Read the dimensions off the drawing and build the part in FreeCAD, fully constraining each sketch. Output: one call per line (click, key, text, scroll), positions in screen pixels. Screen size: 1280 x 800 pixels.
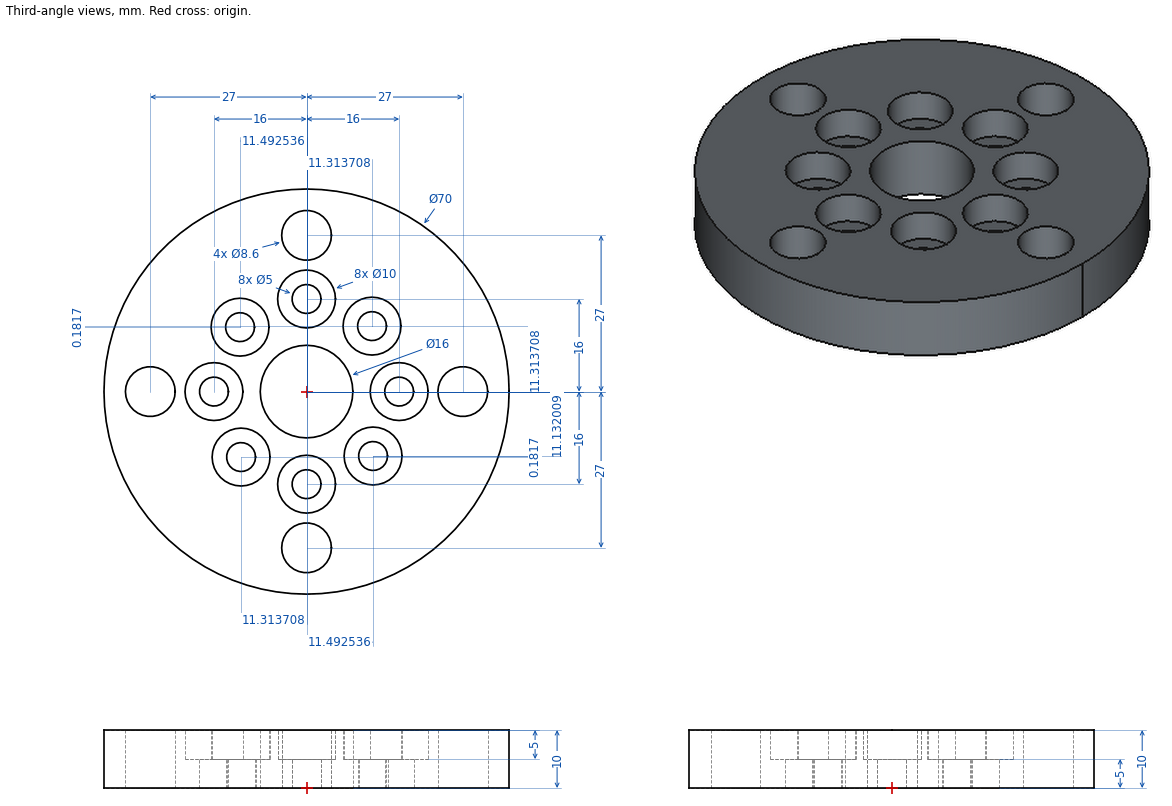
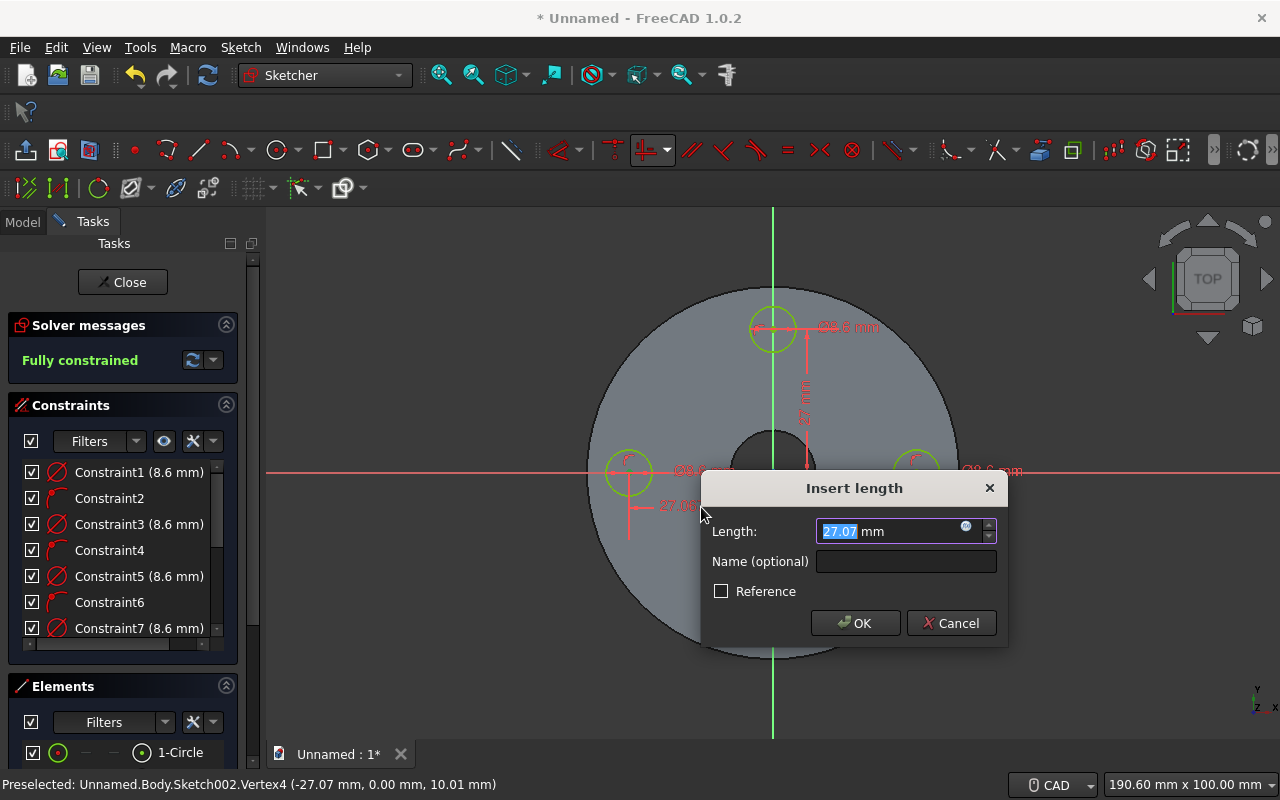
text(27)
key(Return)
key(Escape)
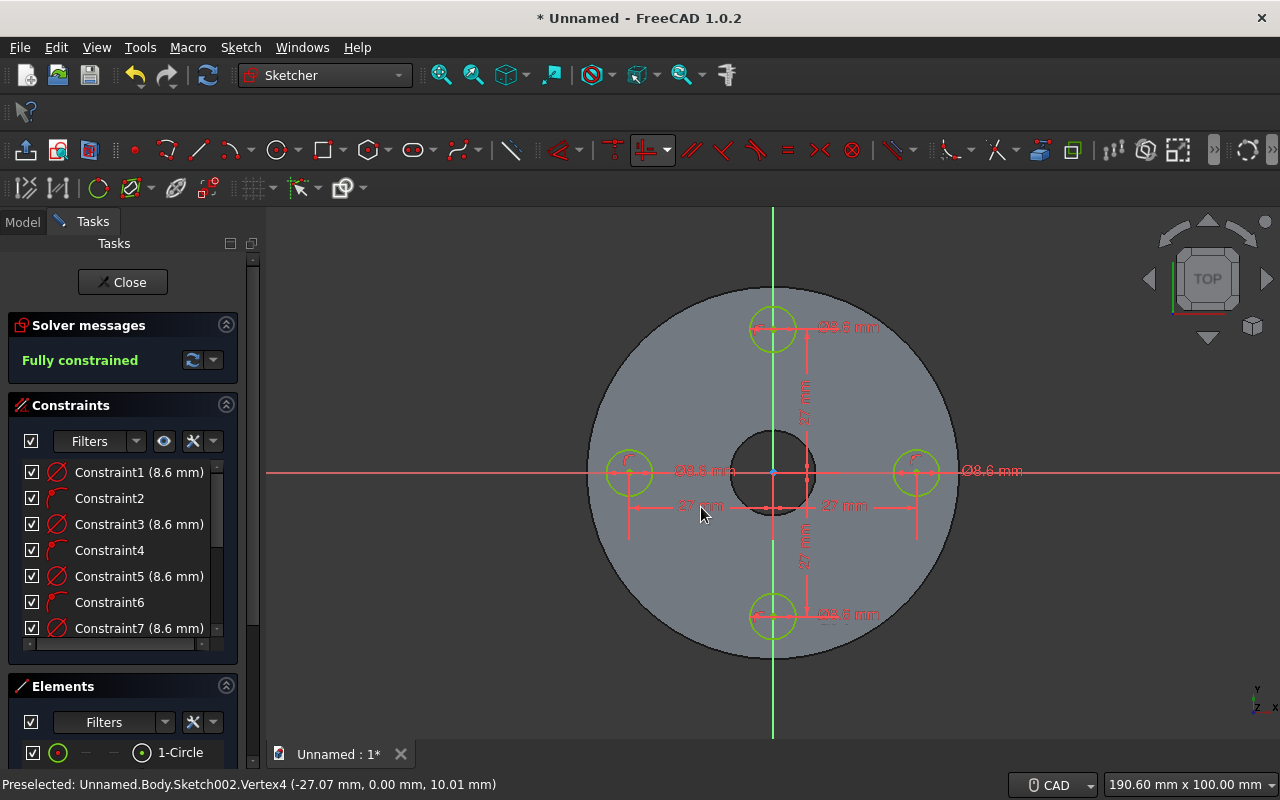
click(123, 282)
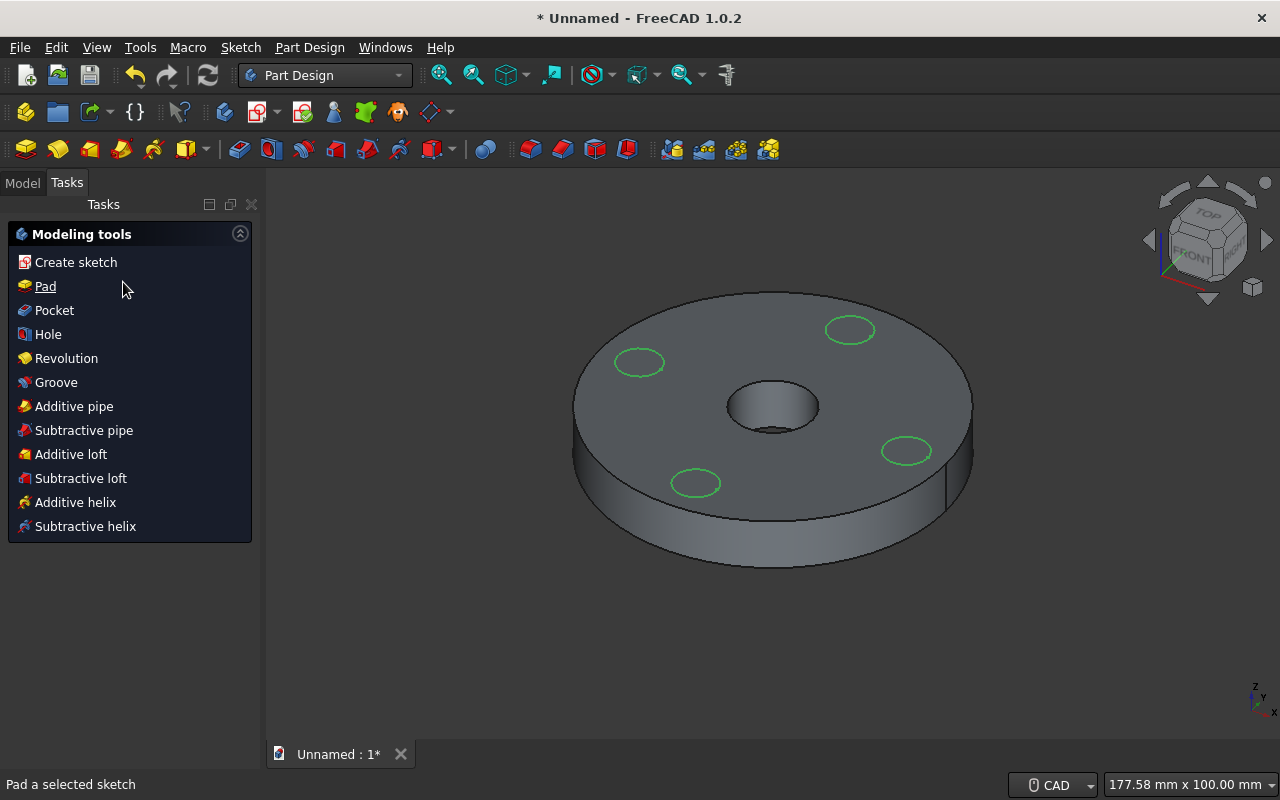
click(240, 150)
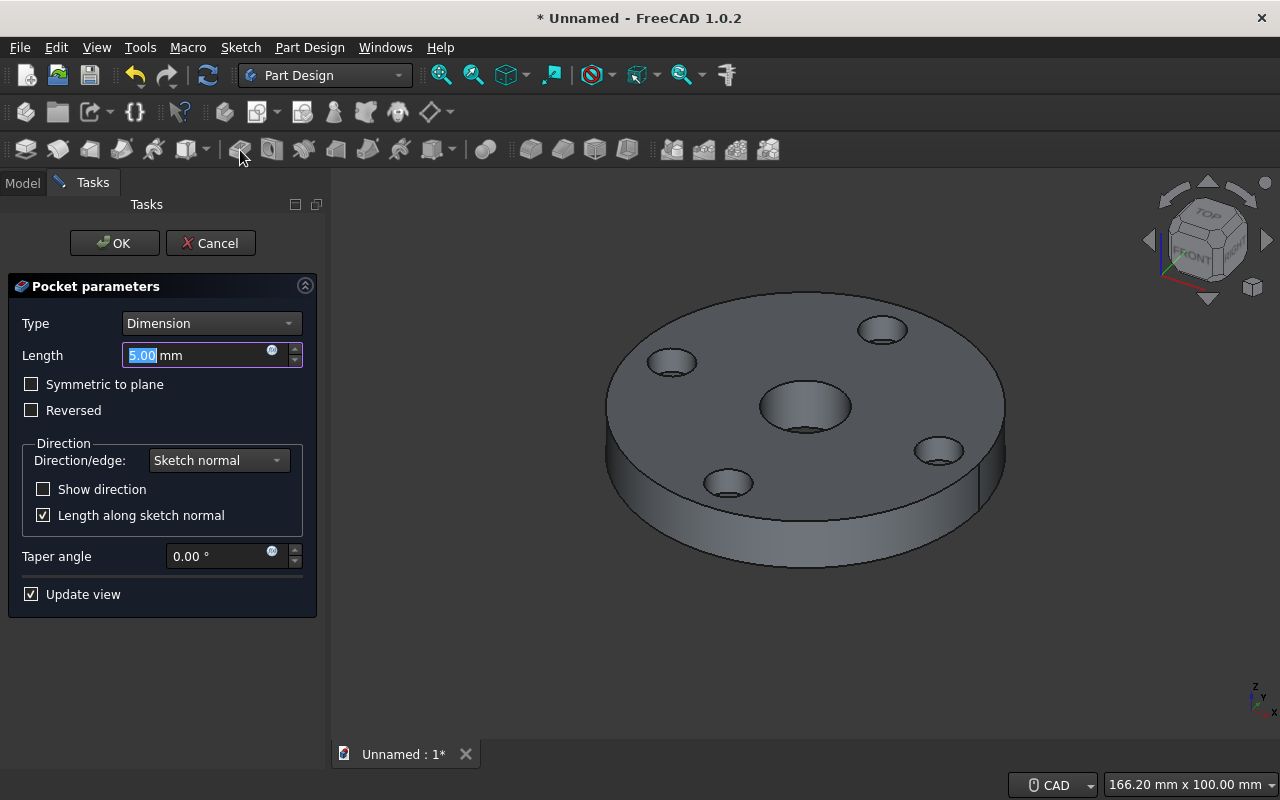
text(10)
key(Tab)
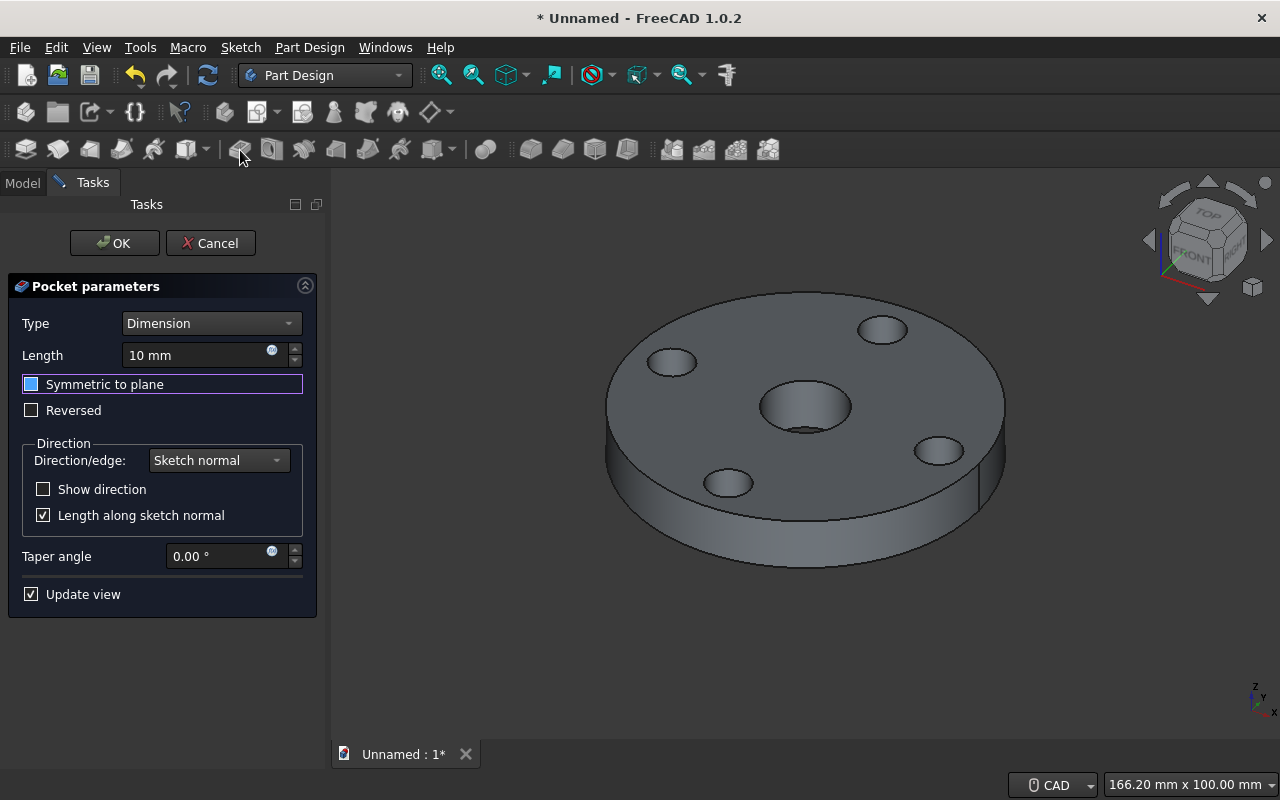
click(115, 243)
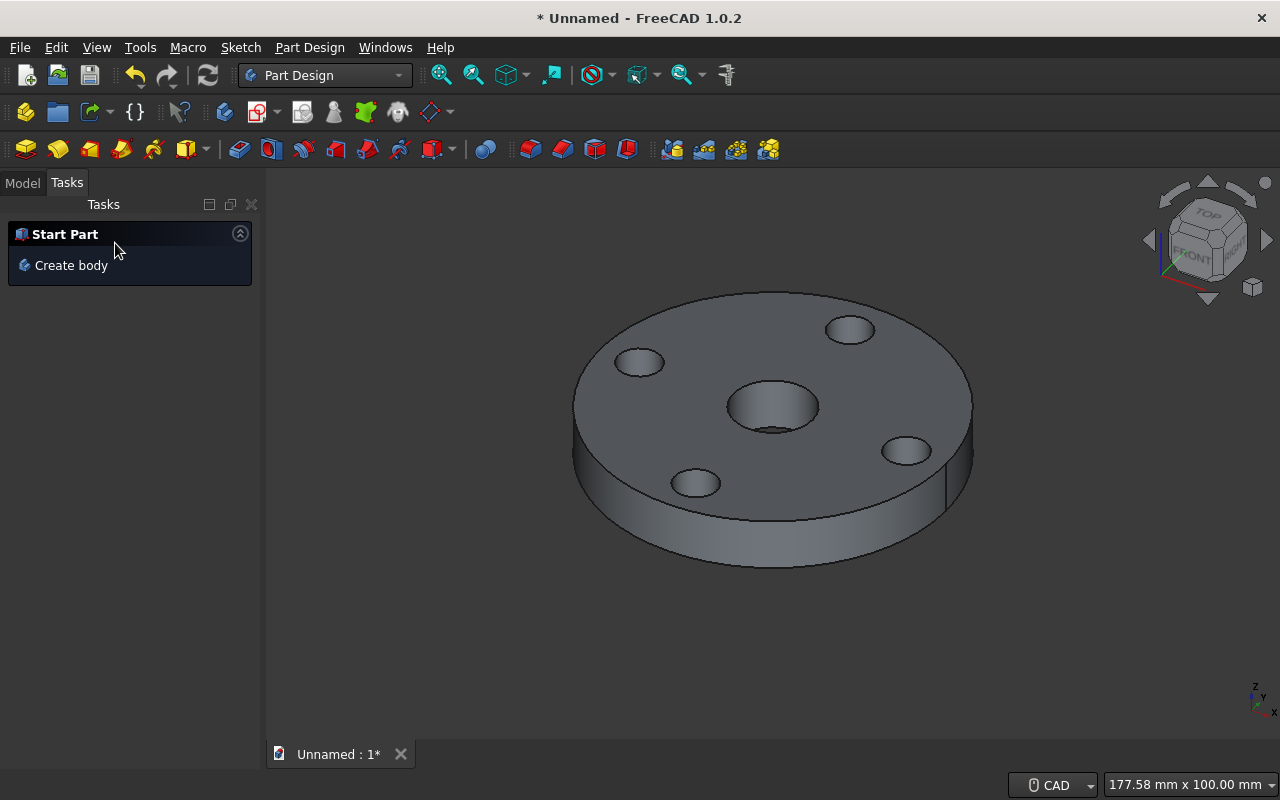
click(666, 446)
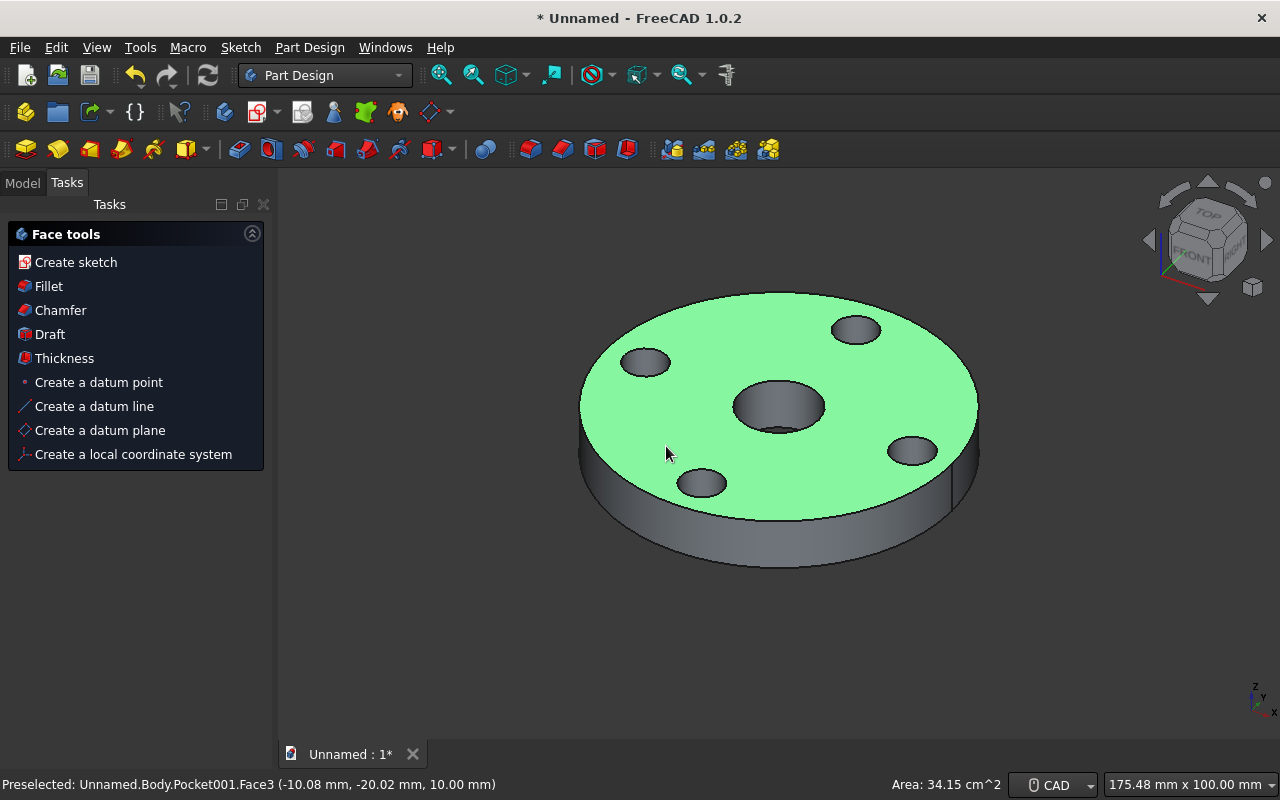
click(258, 112)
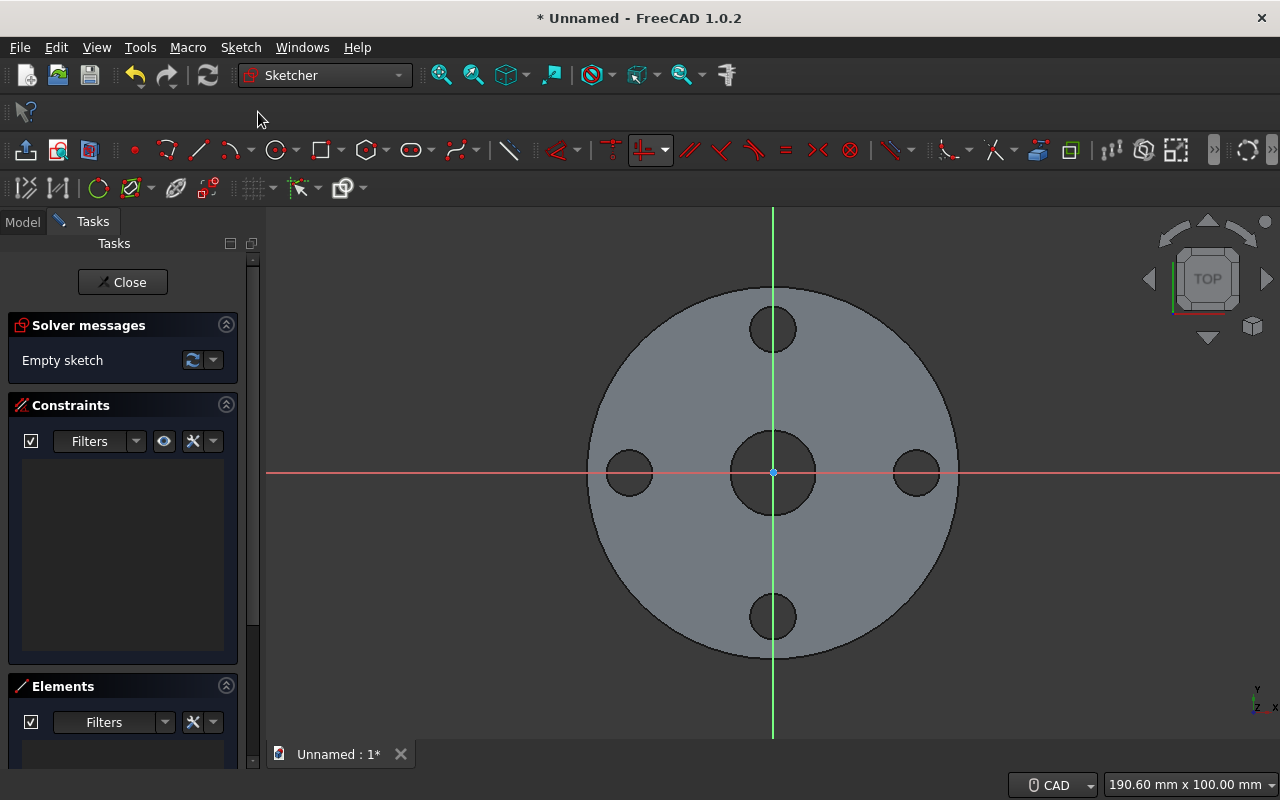
scroll(912, 473, up, 2)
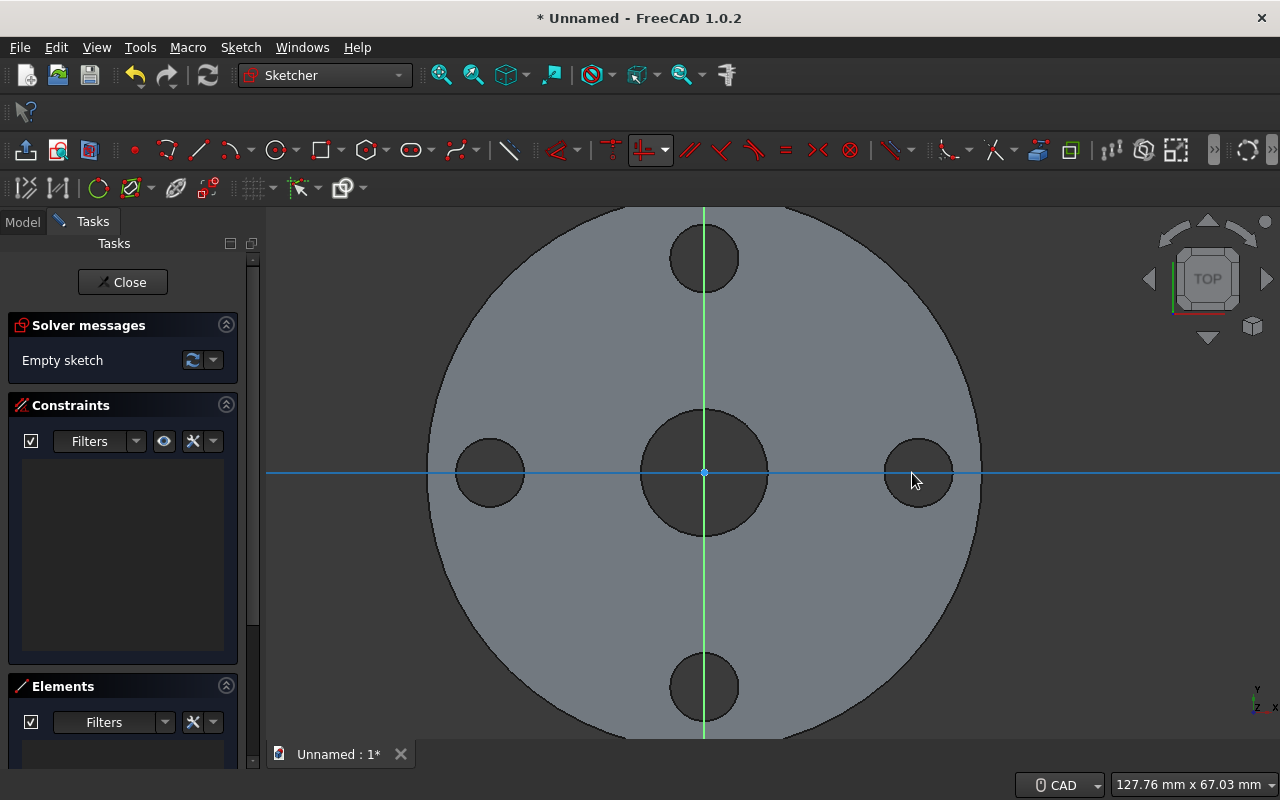
click(276, 150)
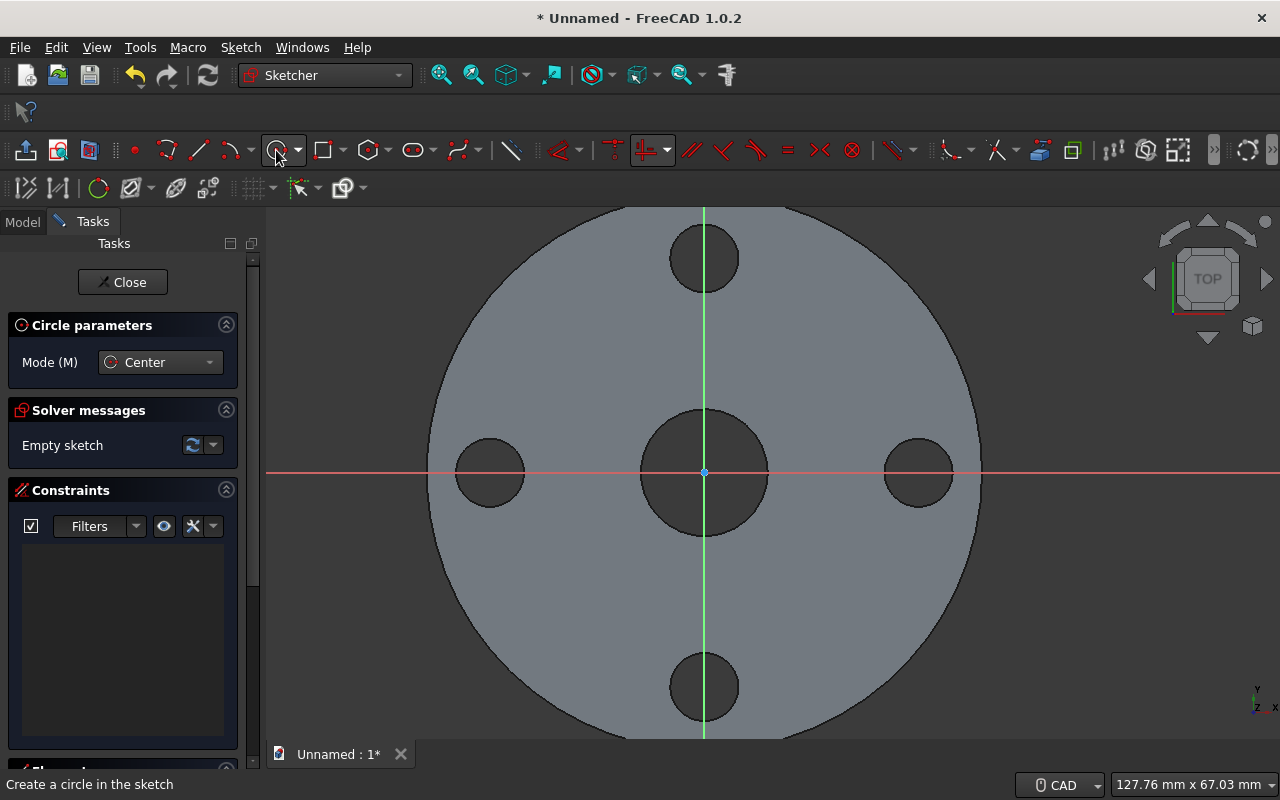
click(704, 346)
move(732, 318)